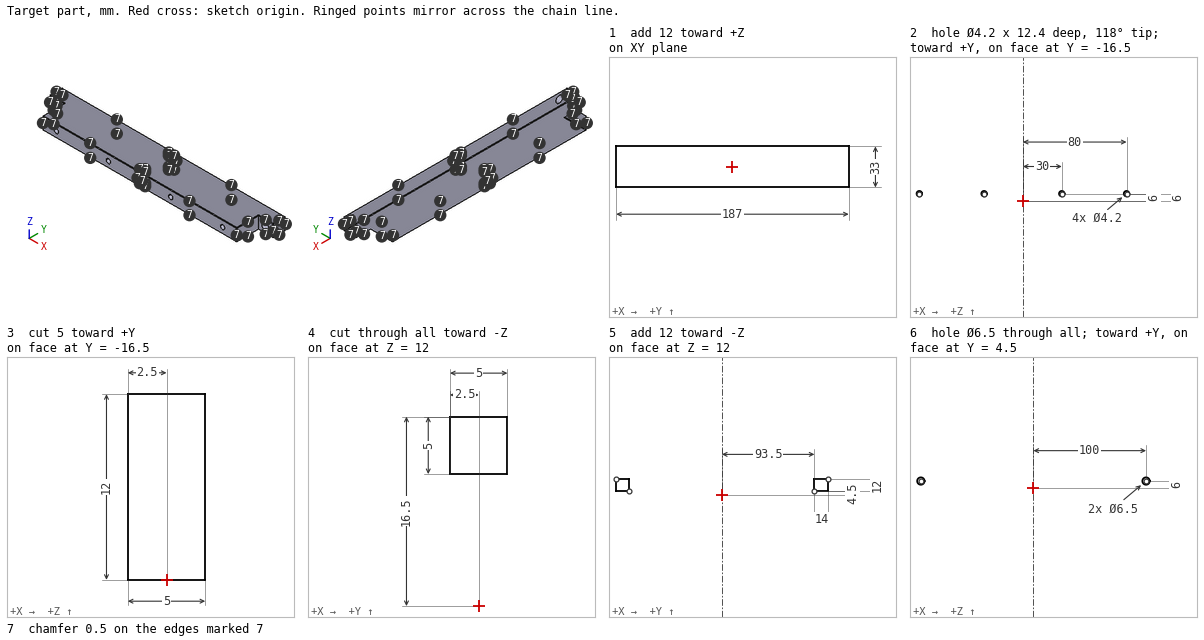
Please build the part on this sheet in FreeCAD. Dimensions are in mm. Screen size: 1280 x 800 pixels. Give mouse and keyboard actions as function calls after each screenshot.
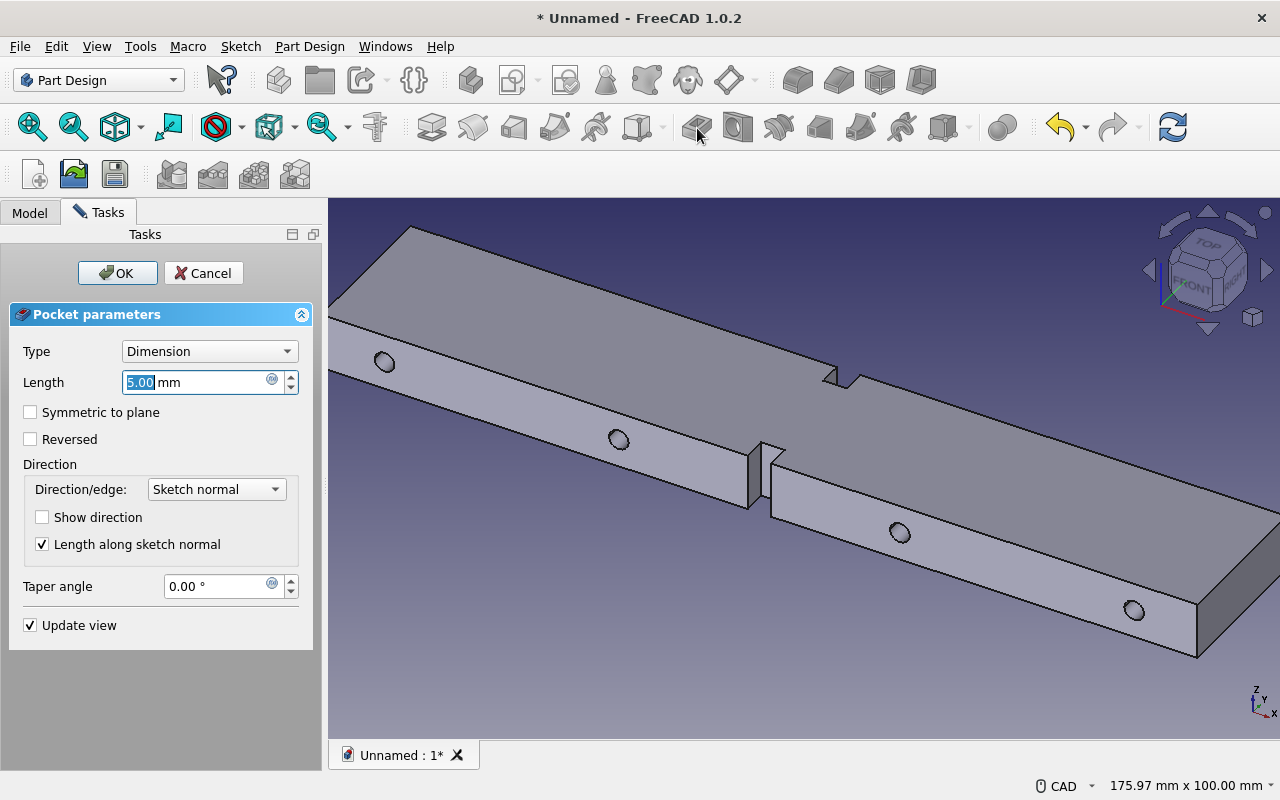
click(210, 352)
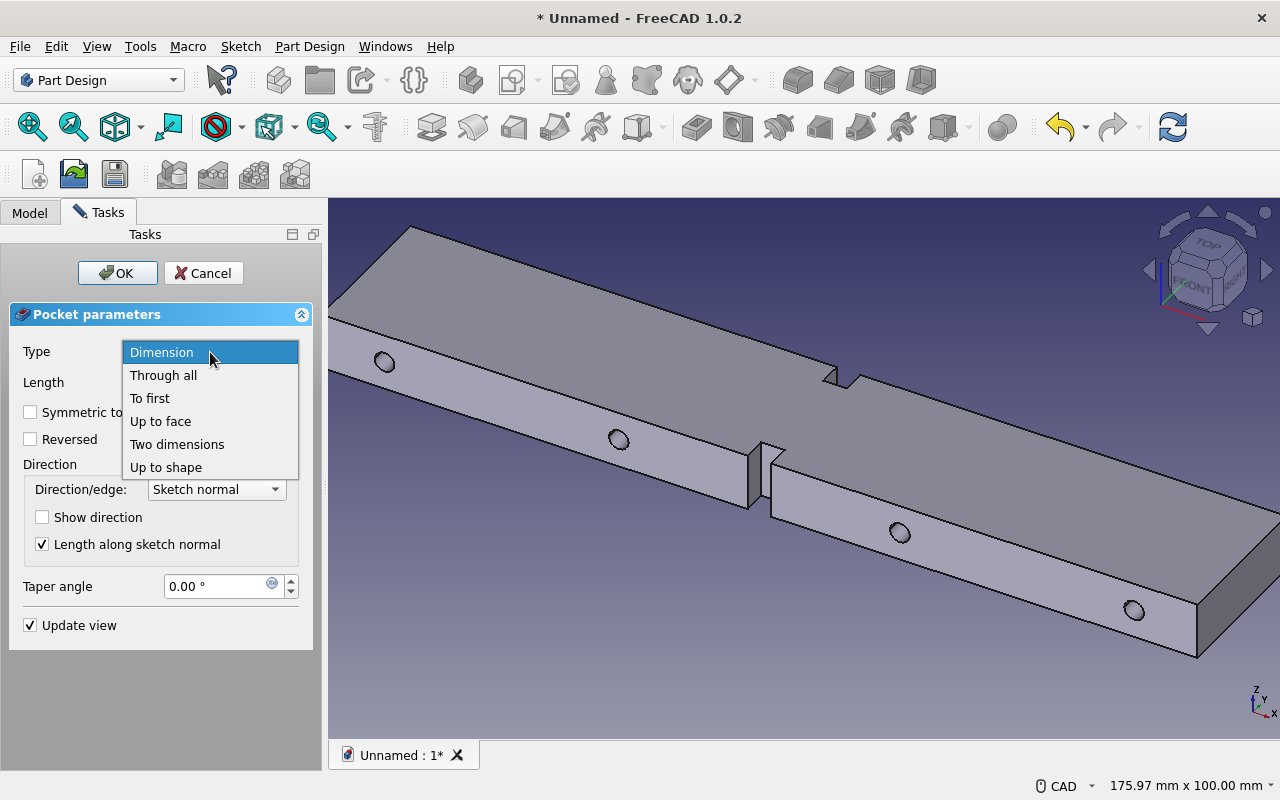
click(208, 376)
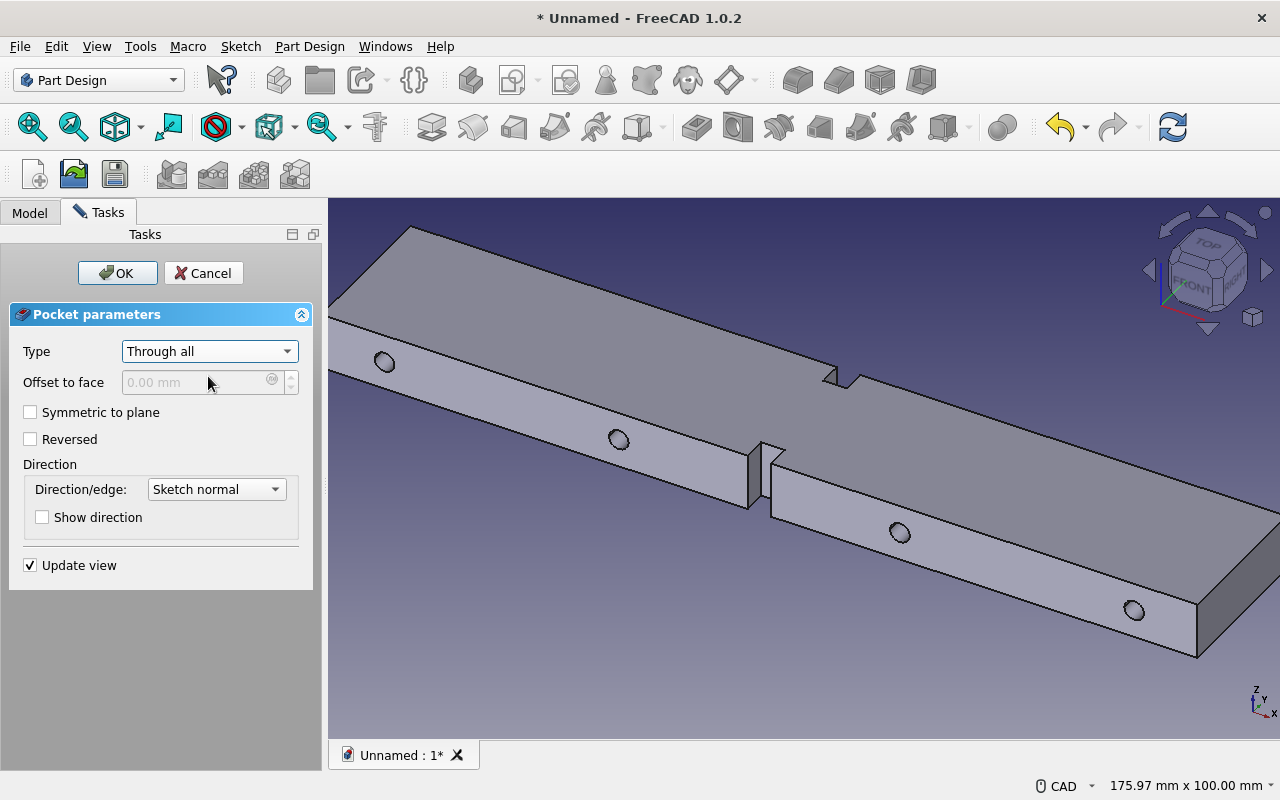
click(118, 273)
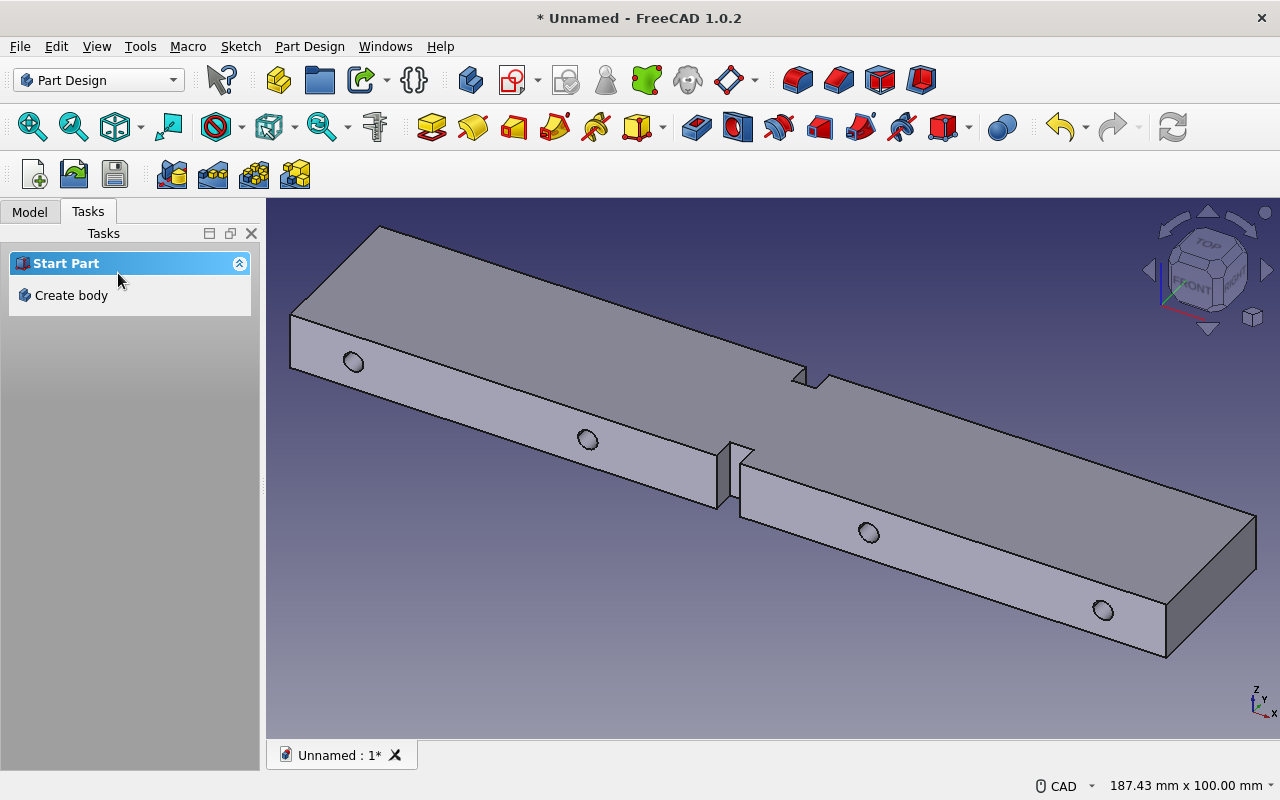
click(1023, 497)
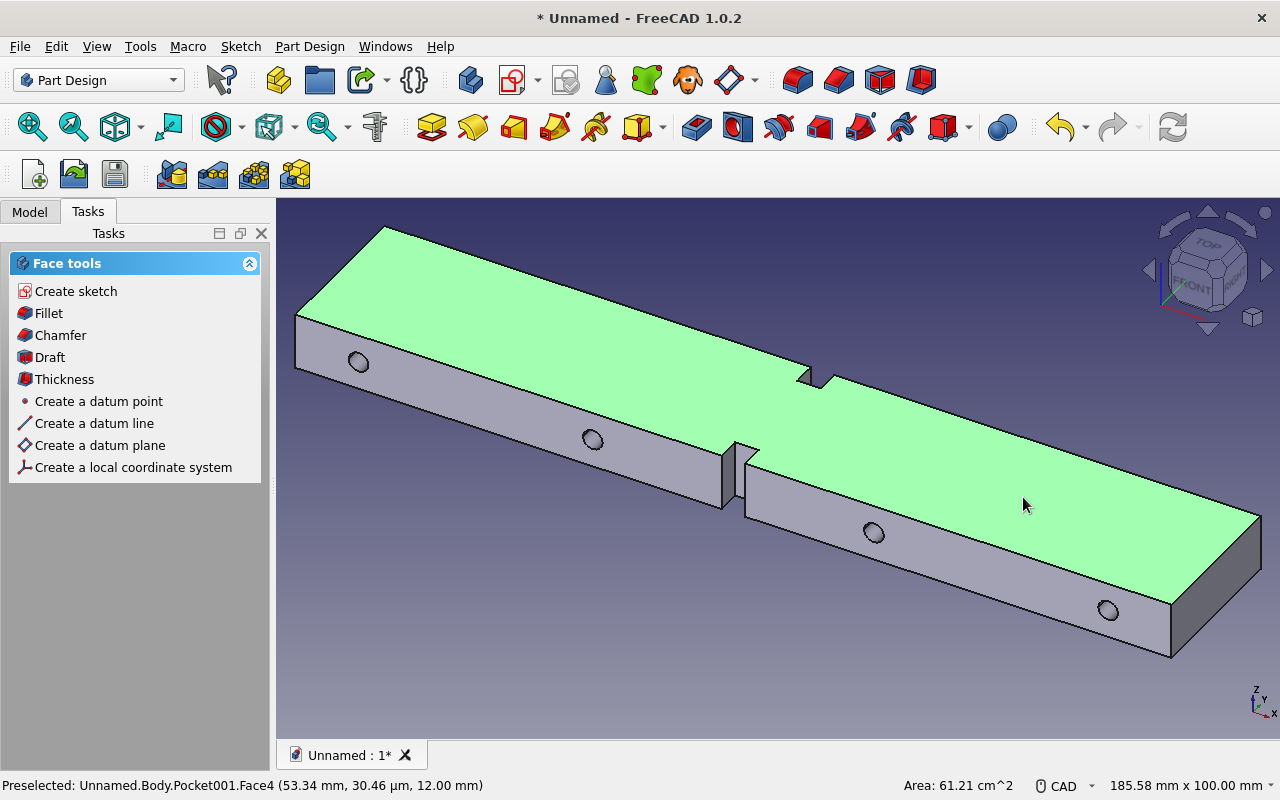
click(512, 80)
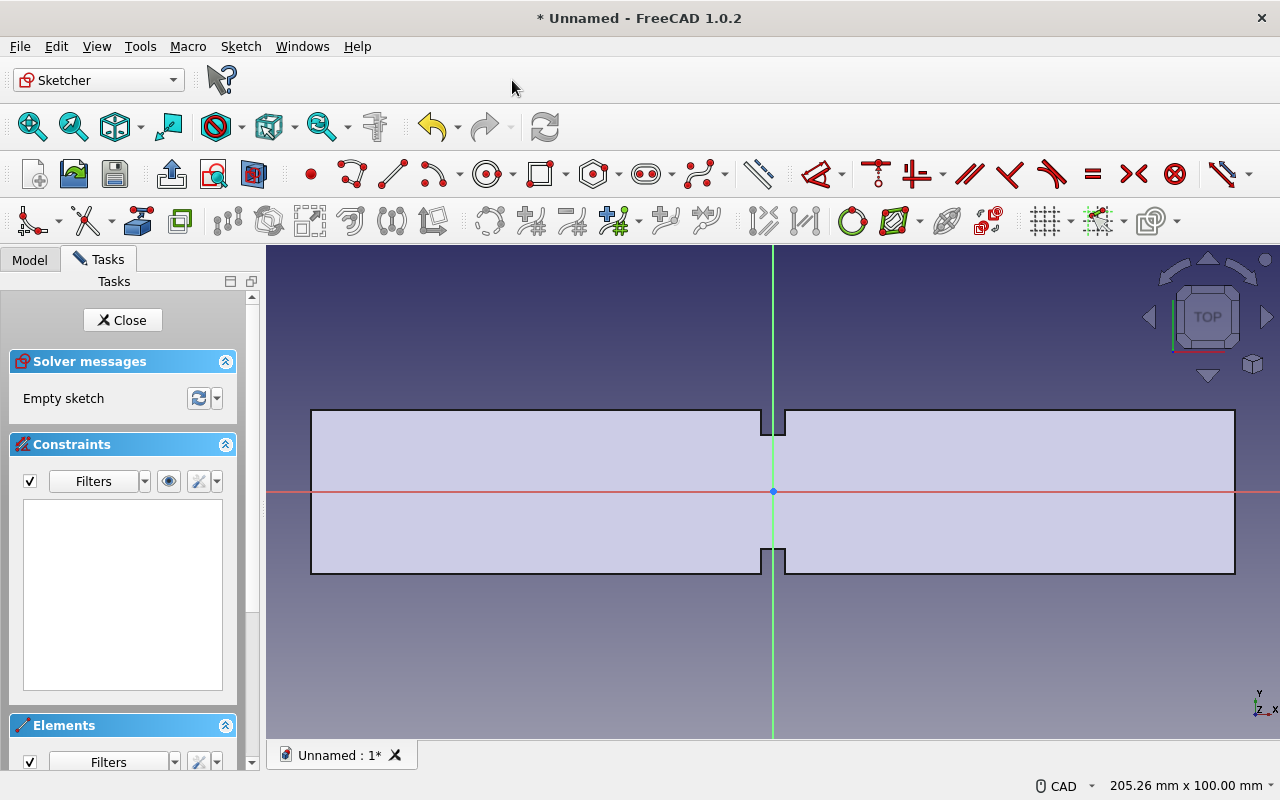
scroll(621, 542, down, 3)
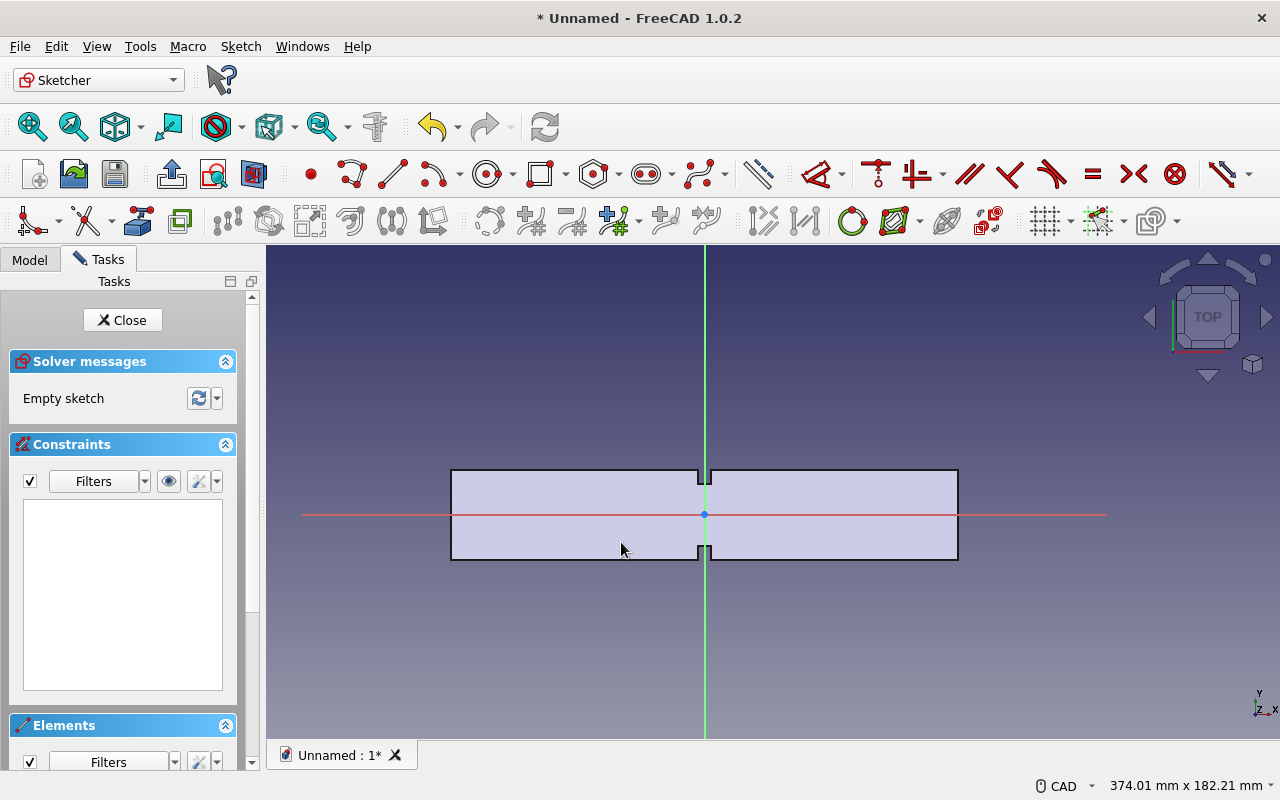
click(540, 174)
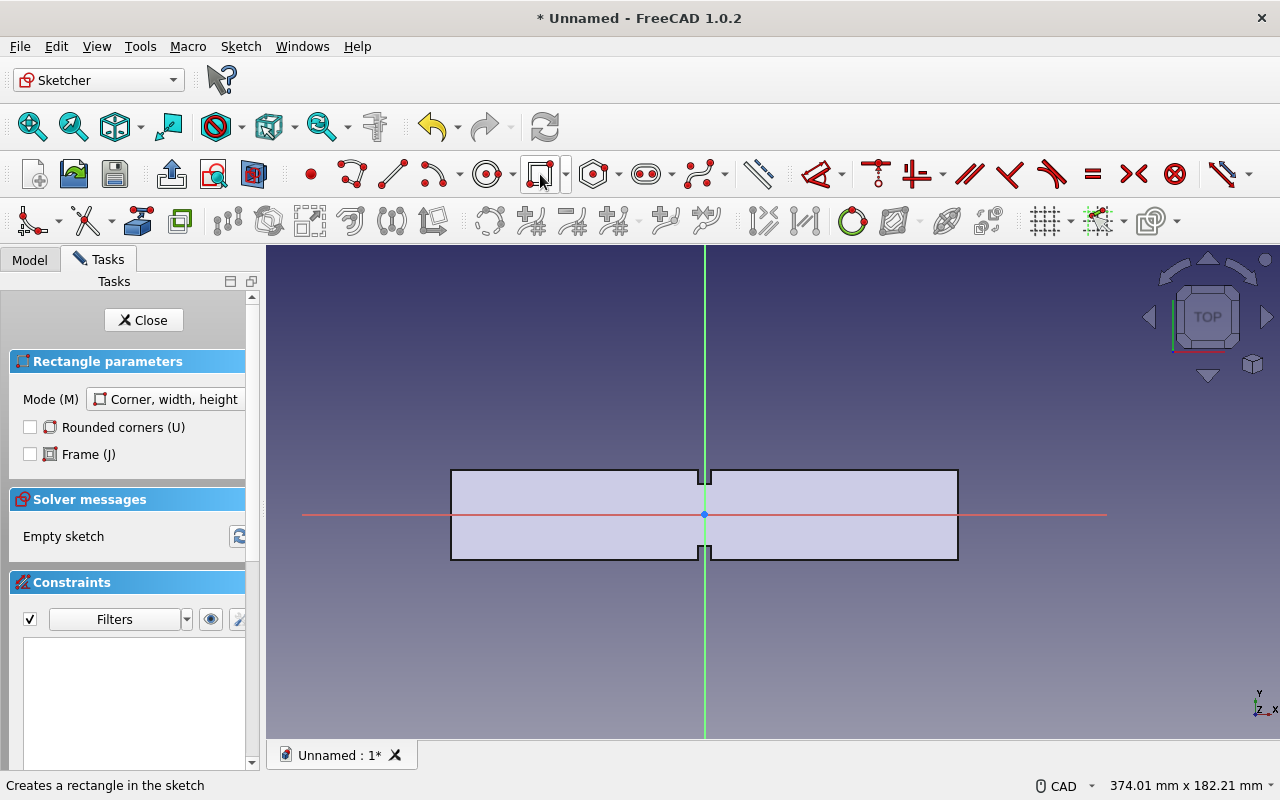
click(958, 470)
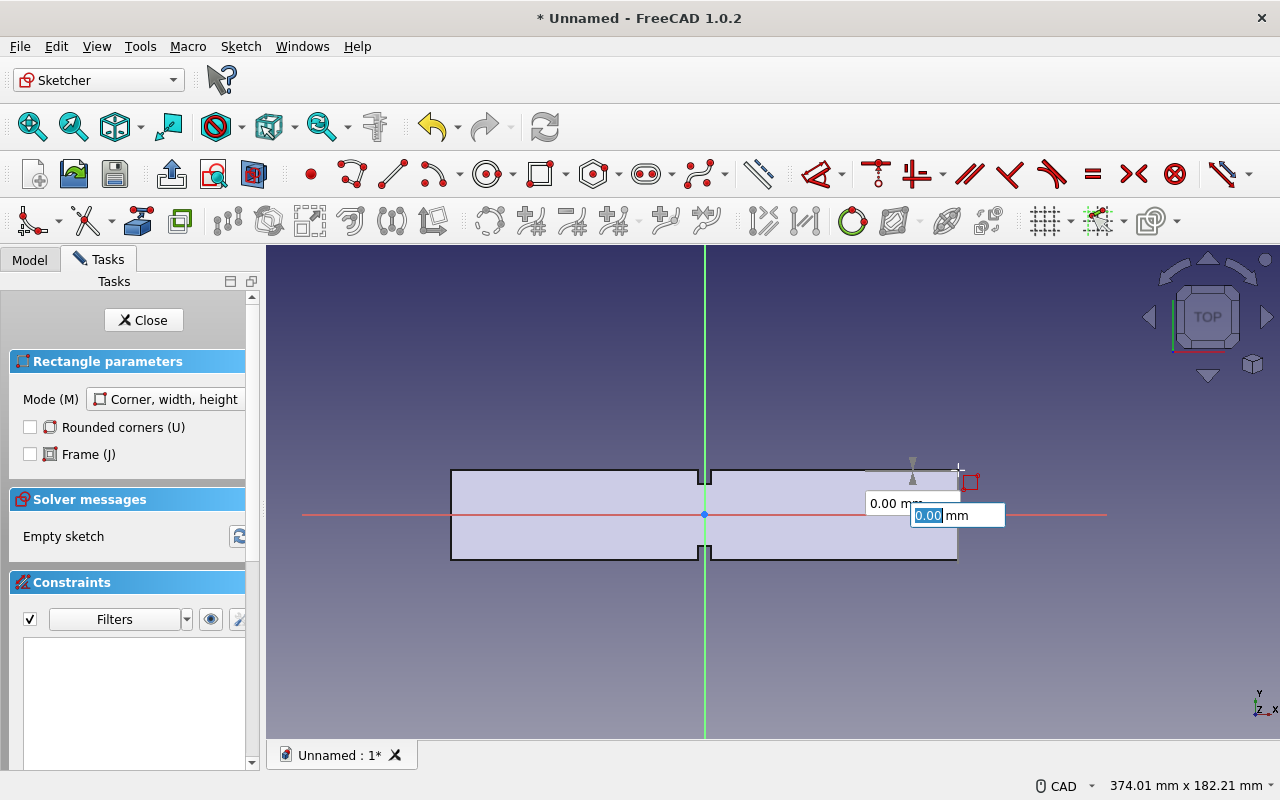
scroll(996, 503, up, 2)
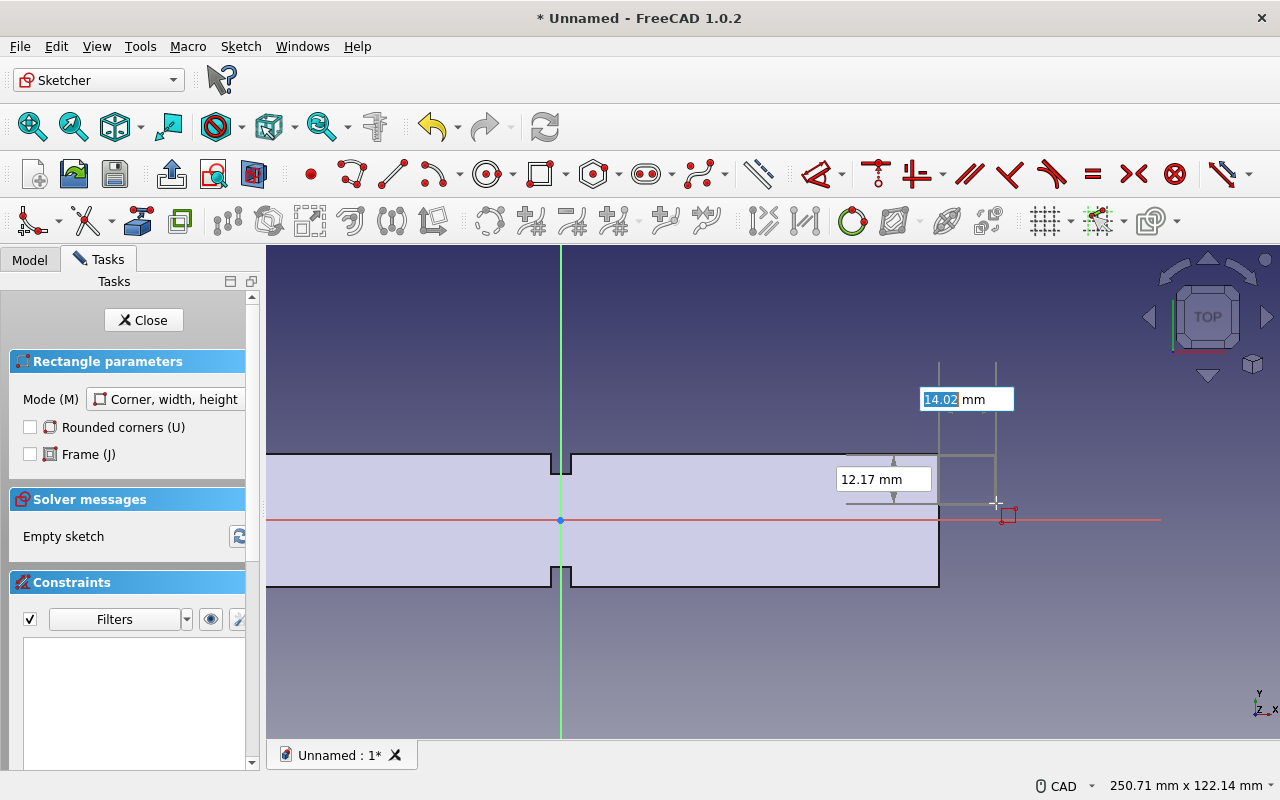
click(996, 502)